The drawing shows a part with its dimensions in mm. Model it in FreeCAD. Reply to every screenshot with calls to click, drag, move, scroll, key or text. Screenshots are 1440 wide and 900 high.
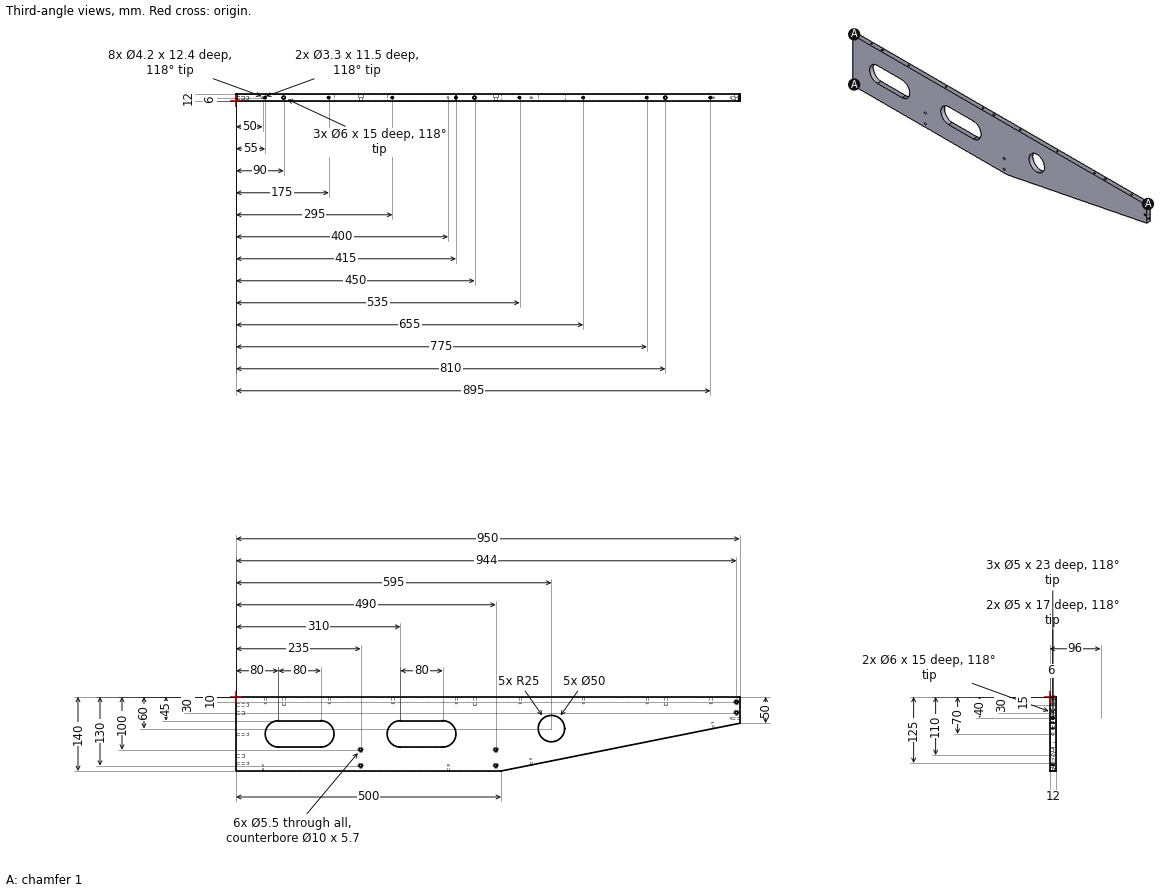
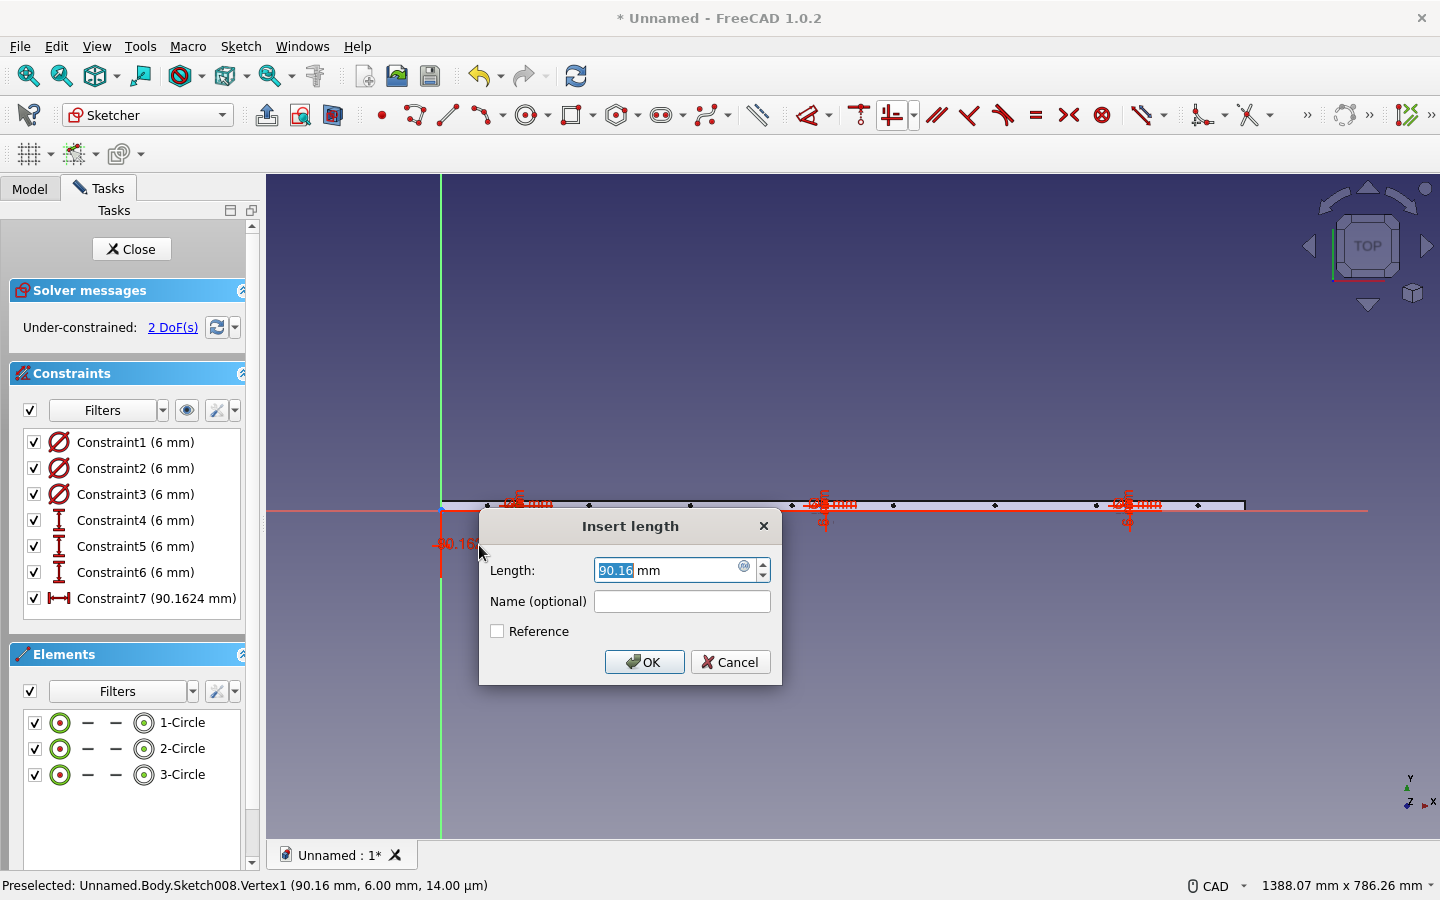
text(90)
key(Return)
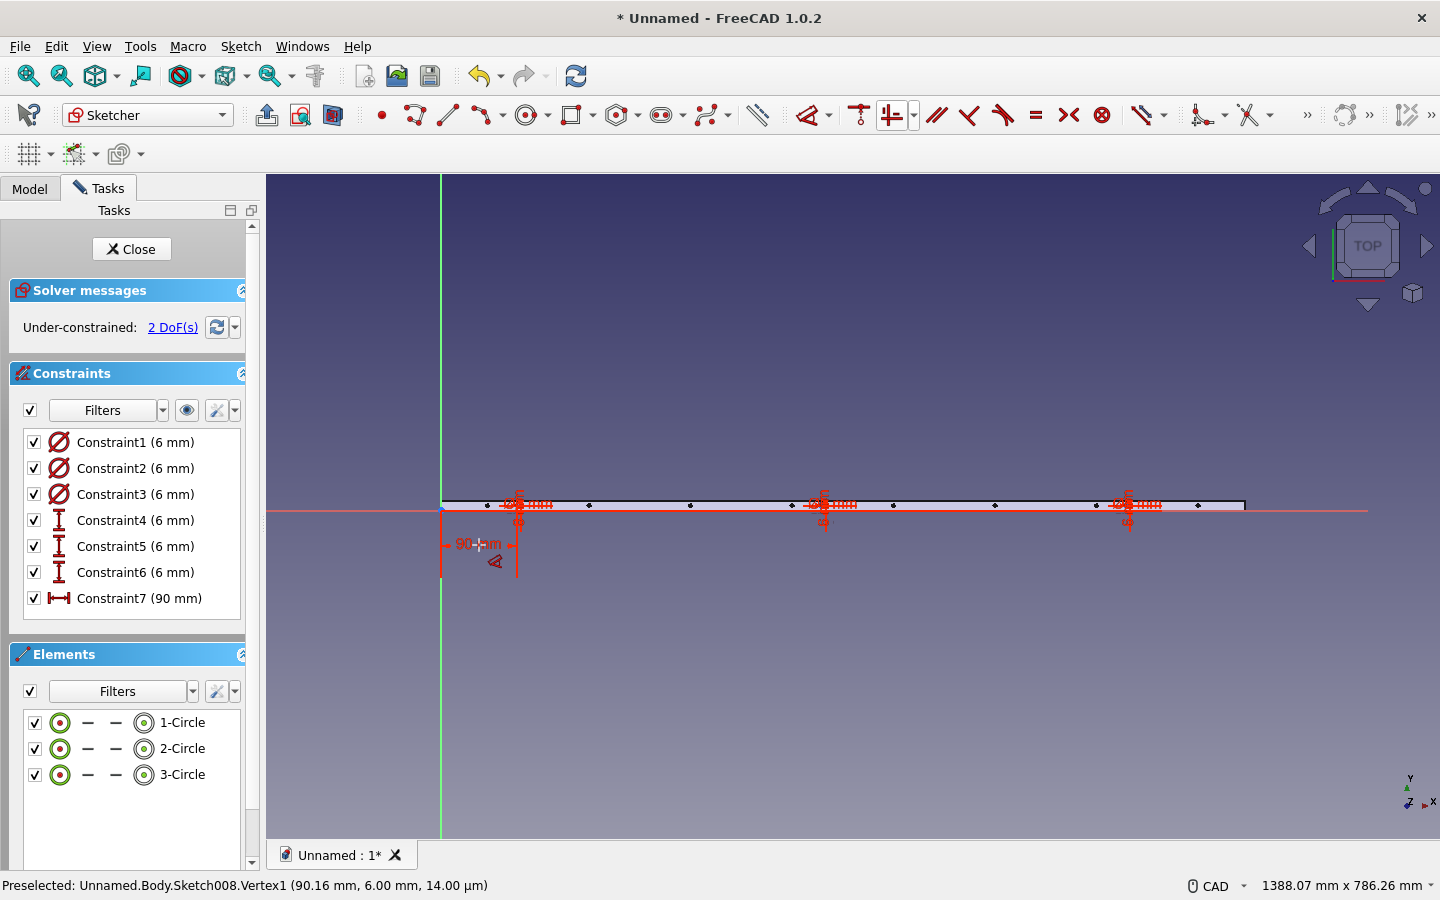
click(822, 506)
click(631, 545)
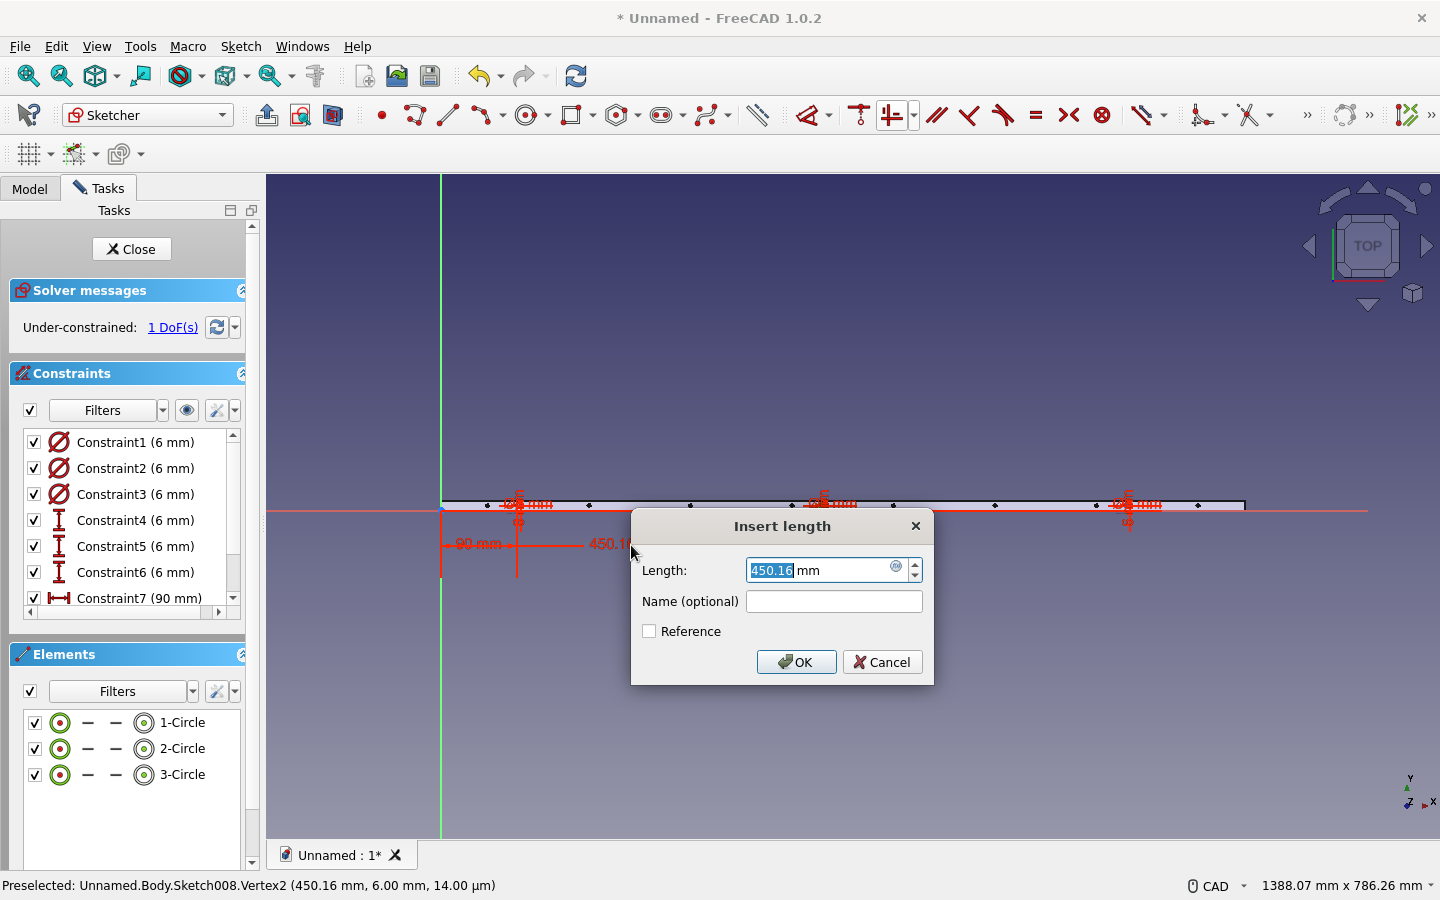
text(450)
key(Return)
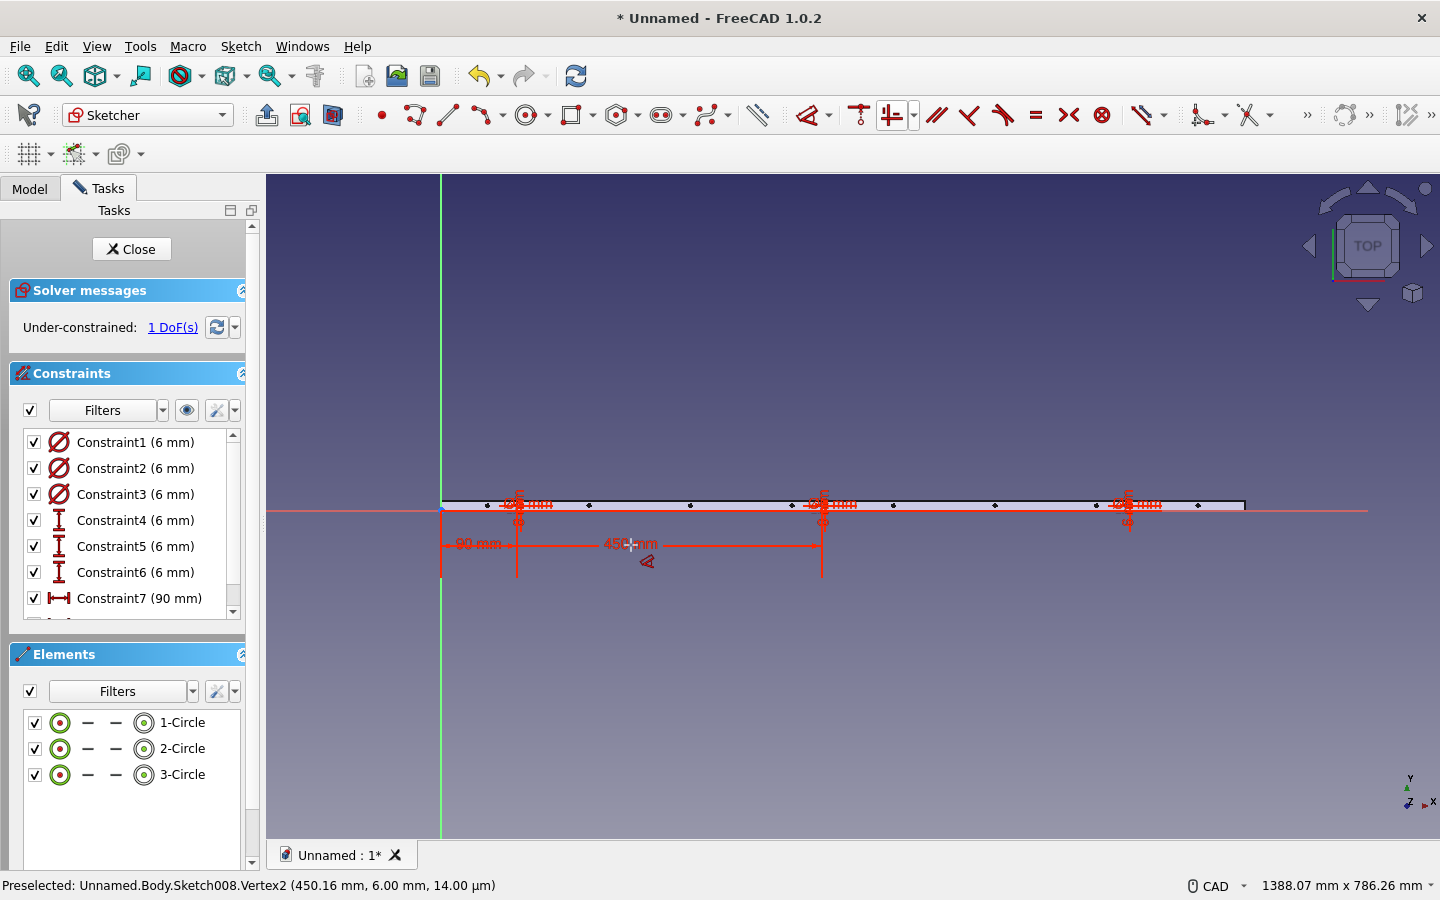
click(1126, 506)
click(784, 545)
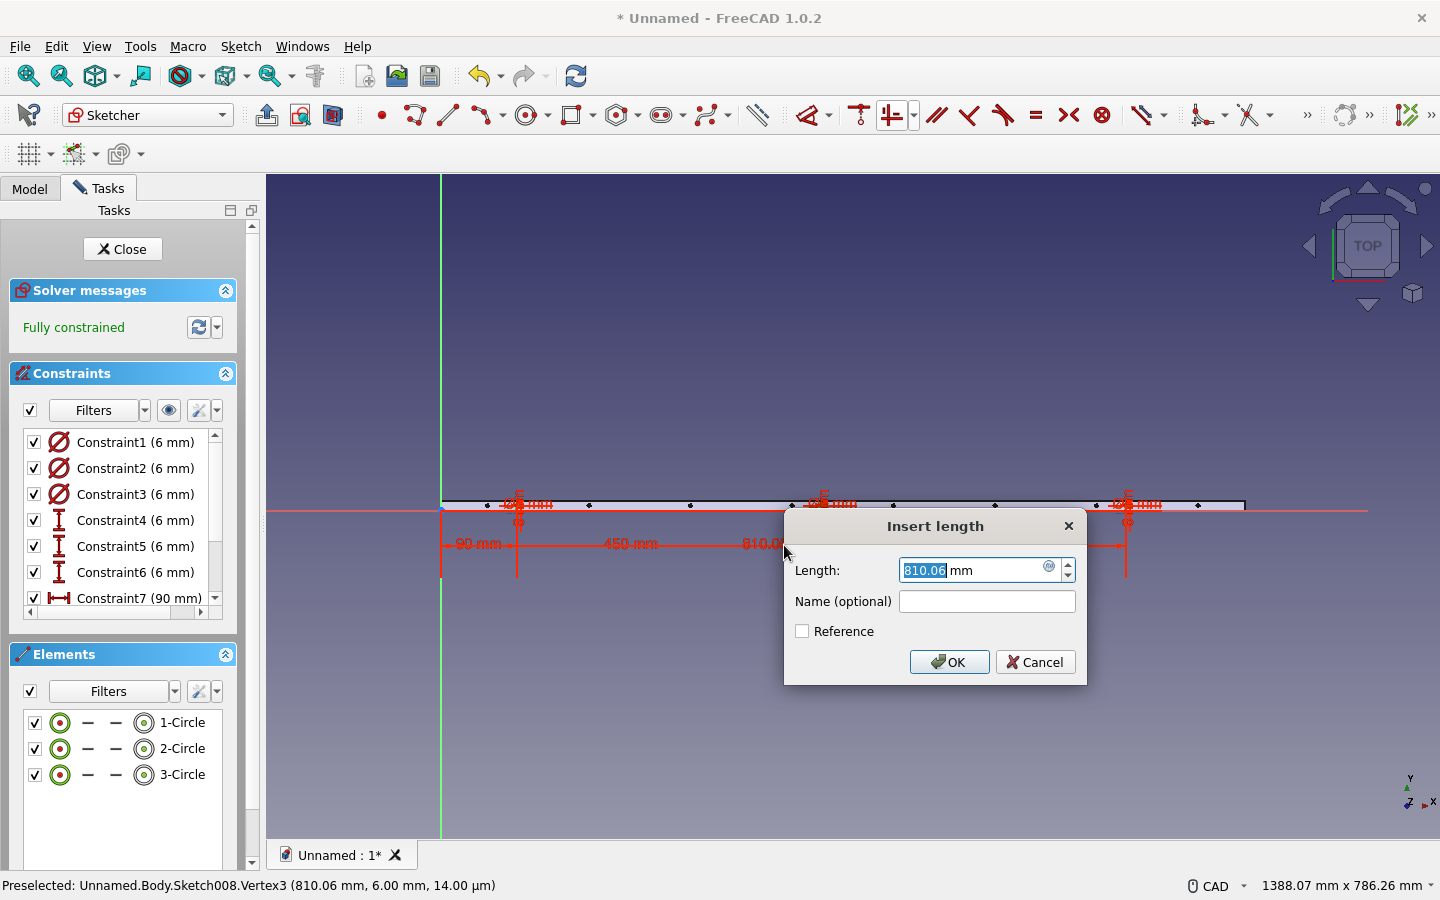
text(810)
key(Return)
key(Escape)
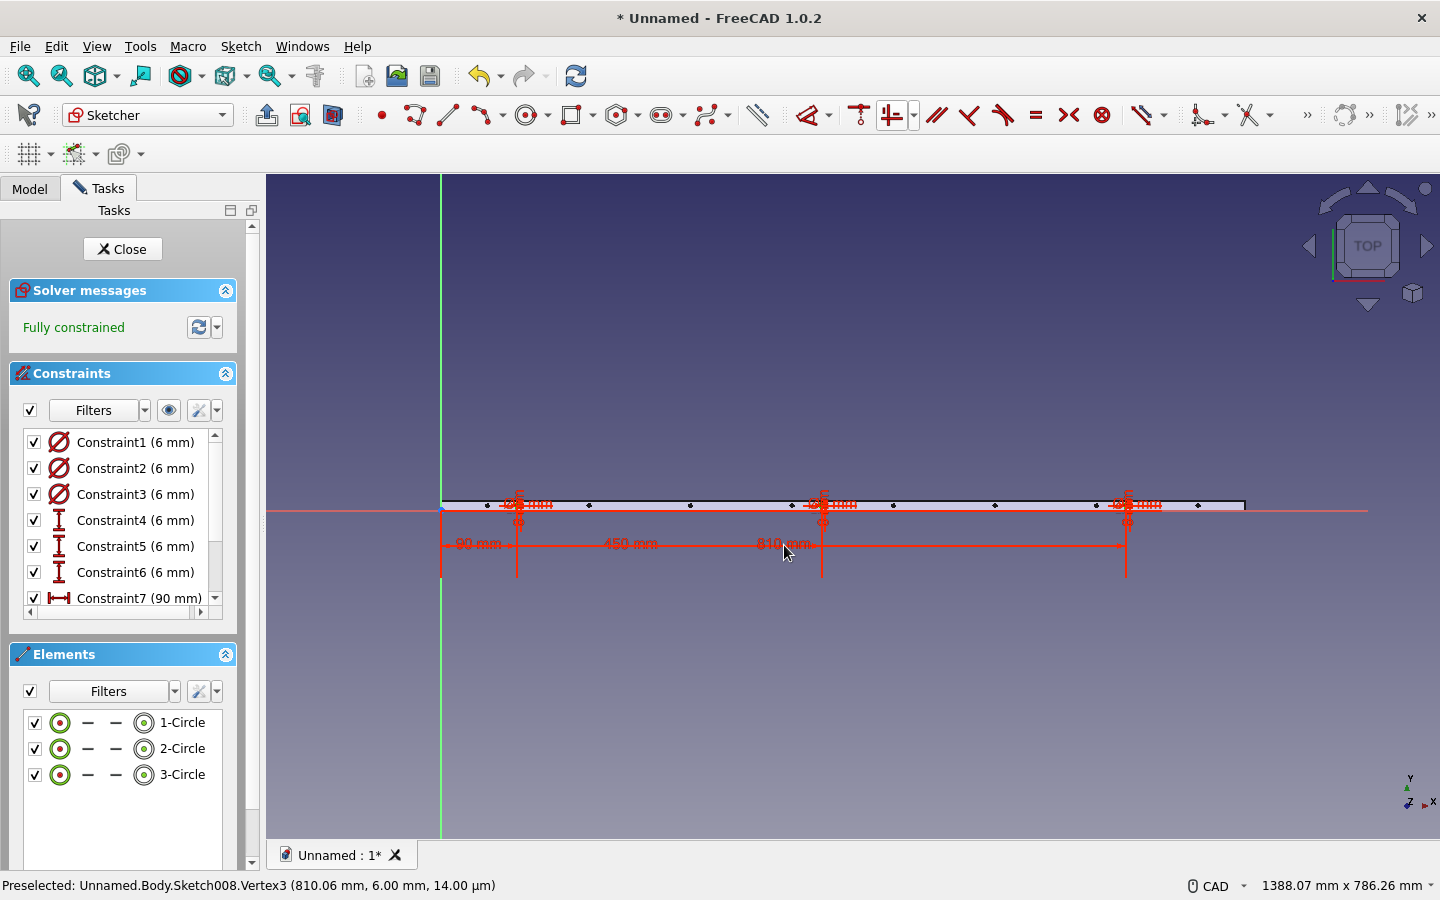
click(123, 249)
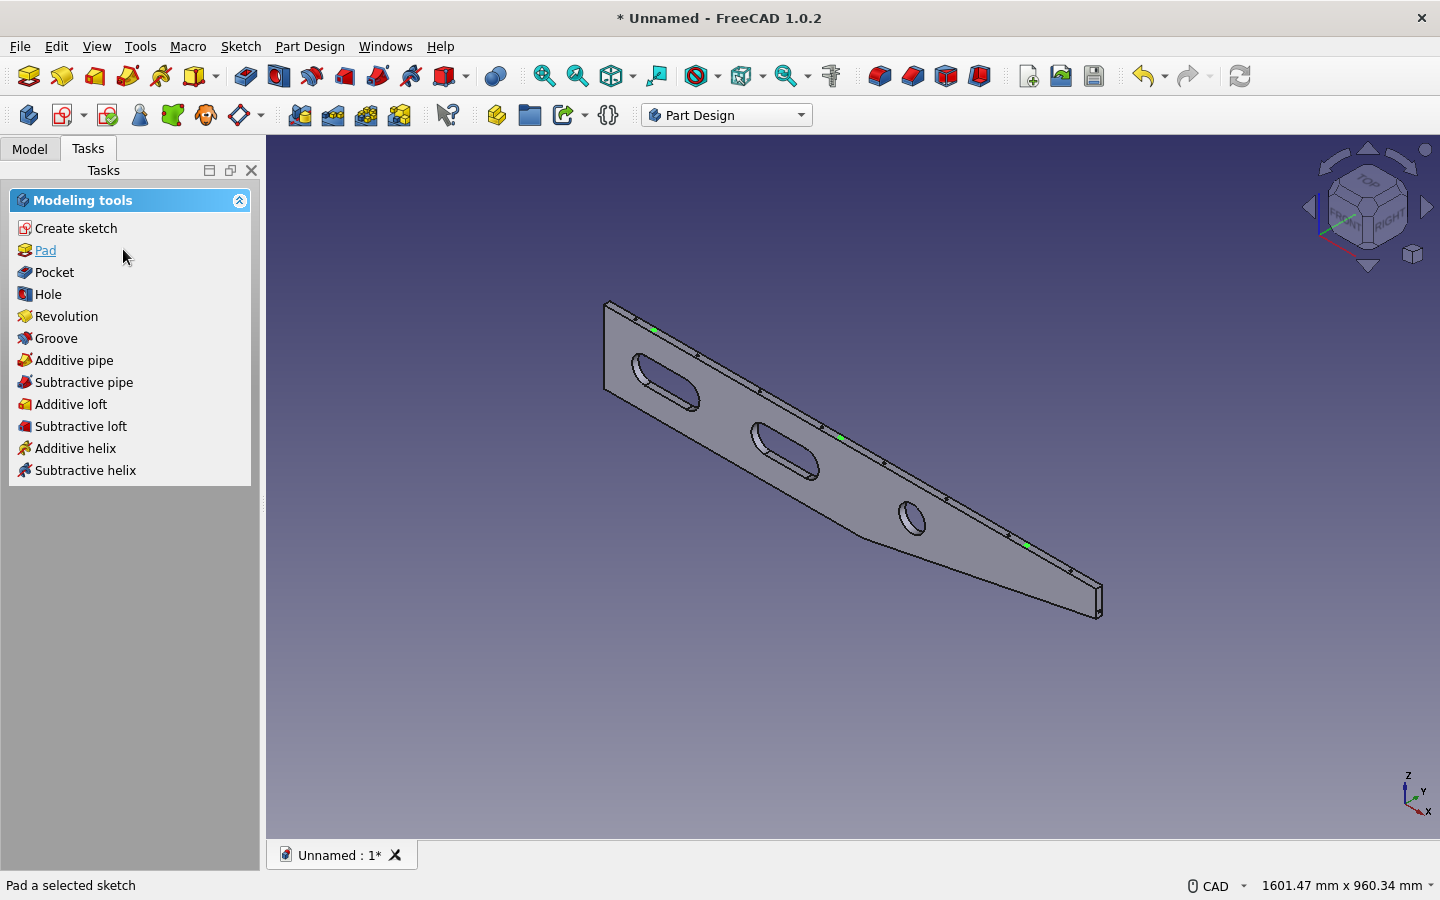
click(279, 76)